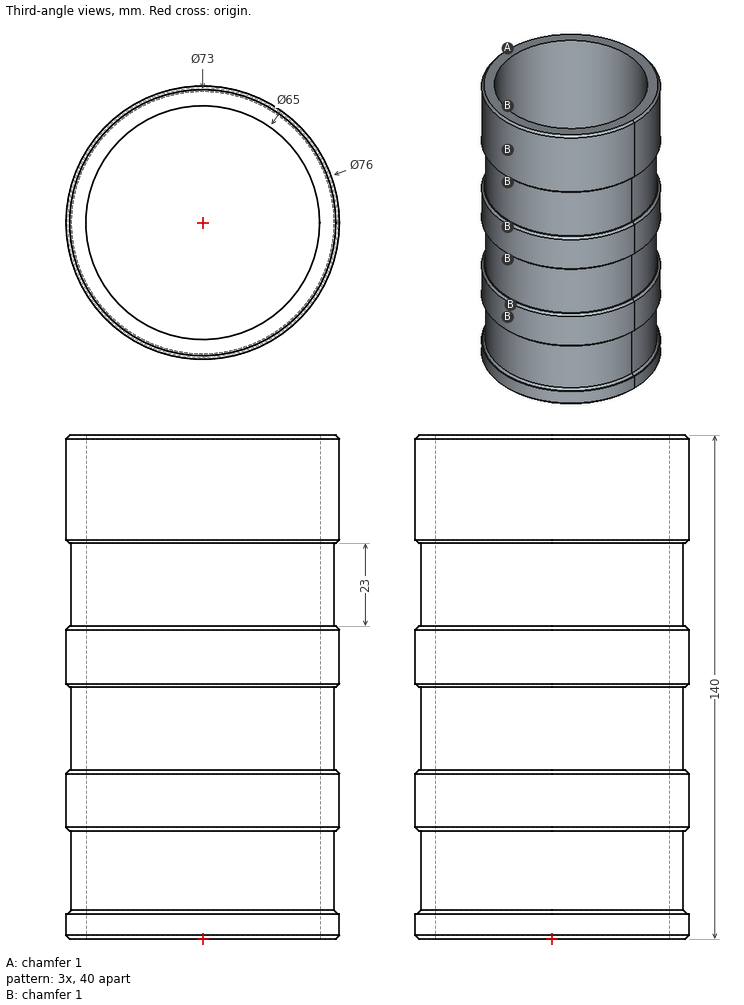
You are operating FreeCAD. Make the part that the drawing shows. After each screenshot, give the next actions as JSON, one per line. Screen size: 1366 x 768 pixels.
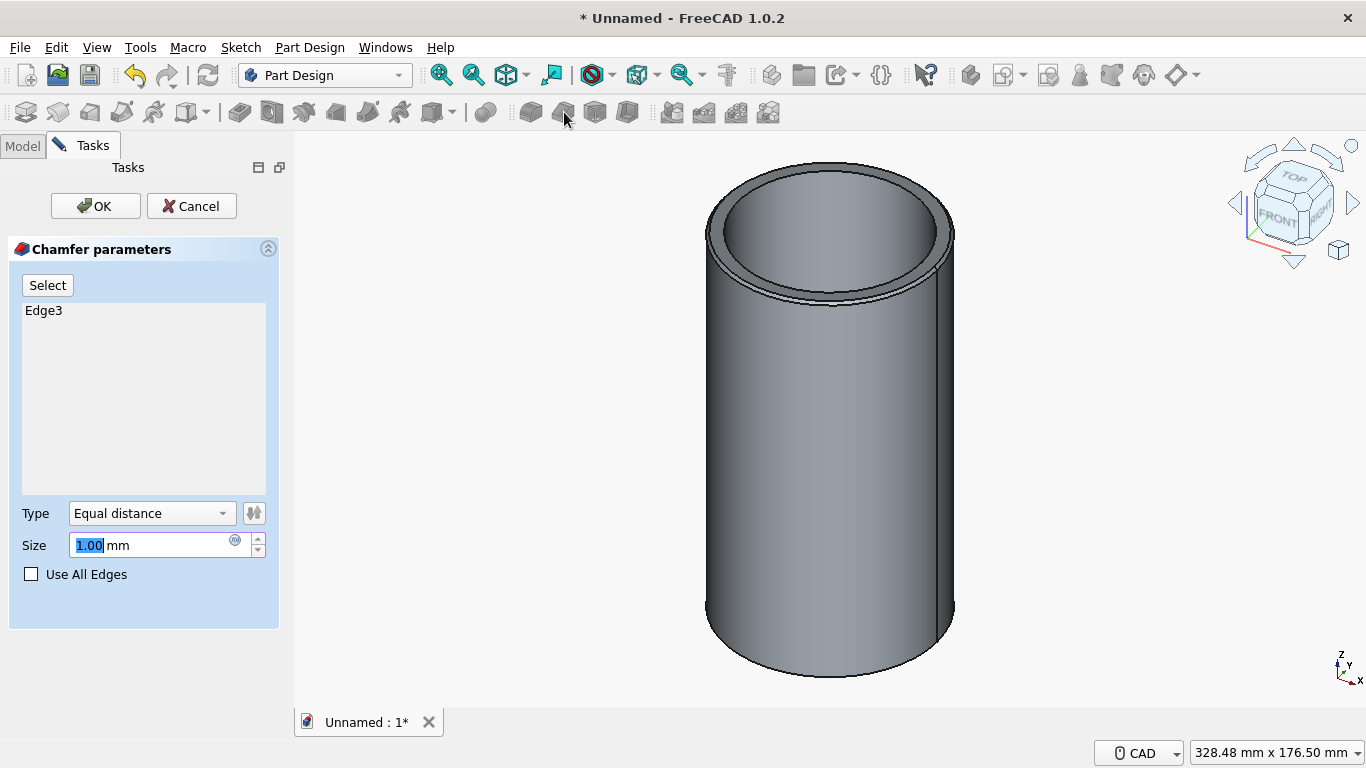
{"action": "type", "text": "1"}
{"action": "key", "text": "Tab"}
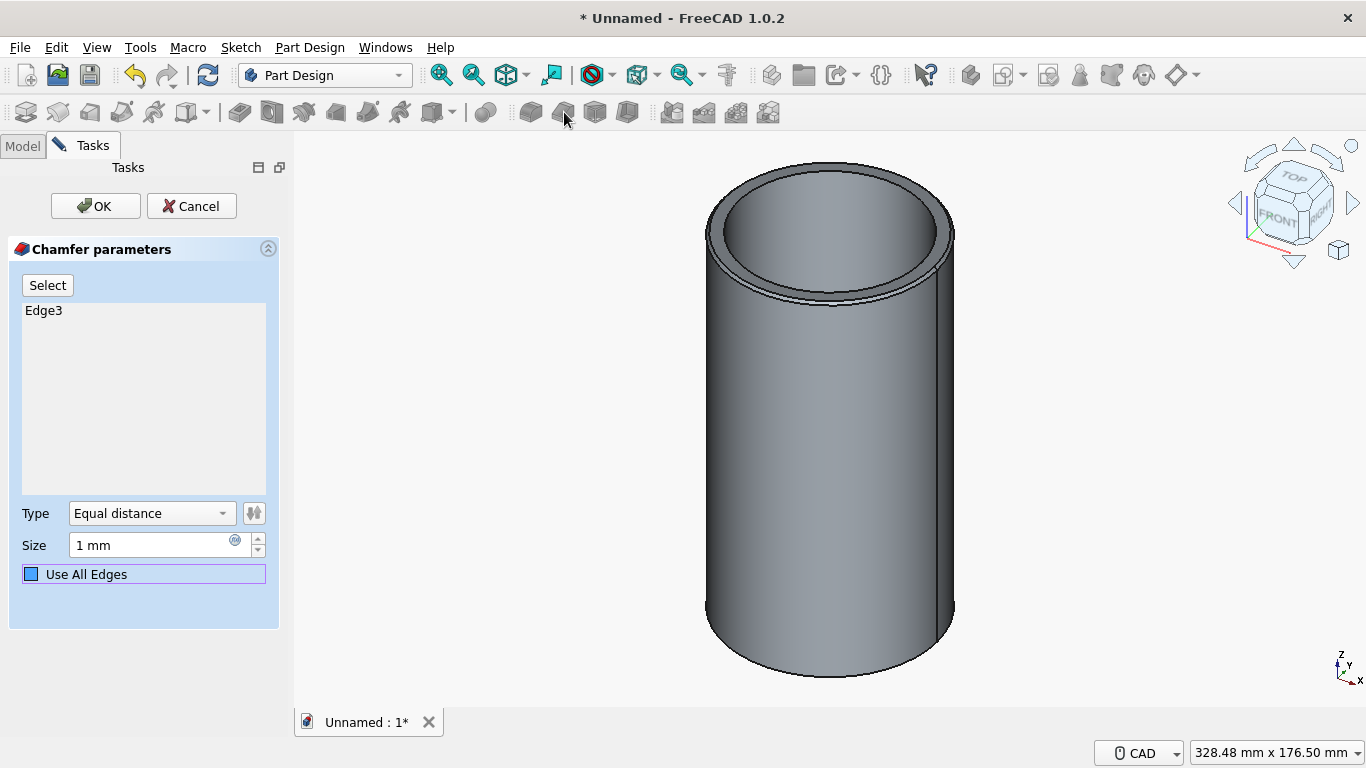
{"action": "left_click", "coordinate": [96, 206]}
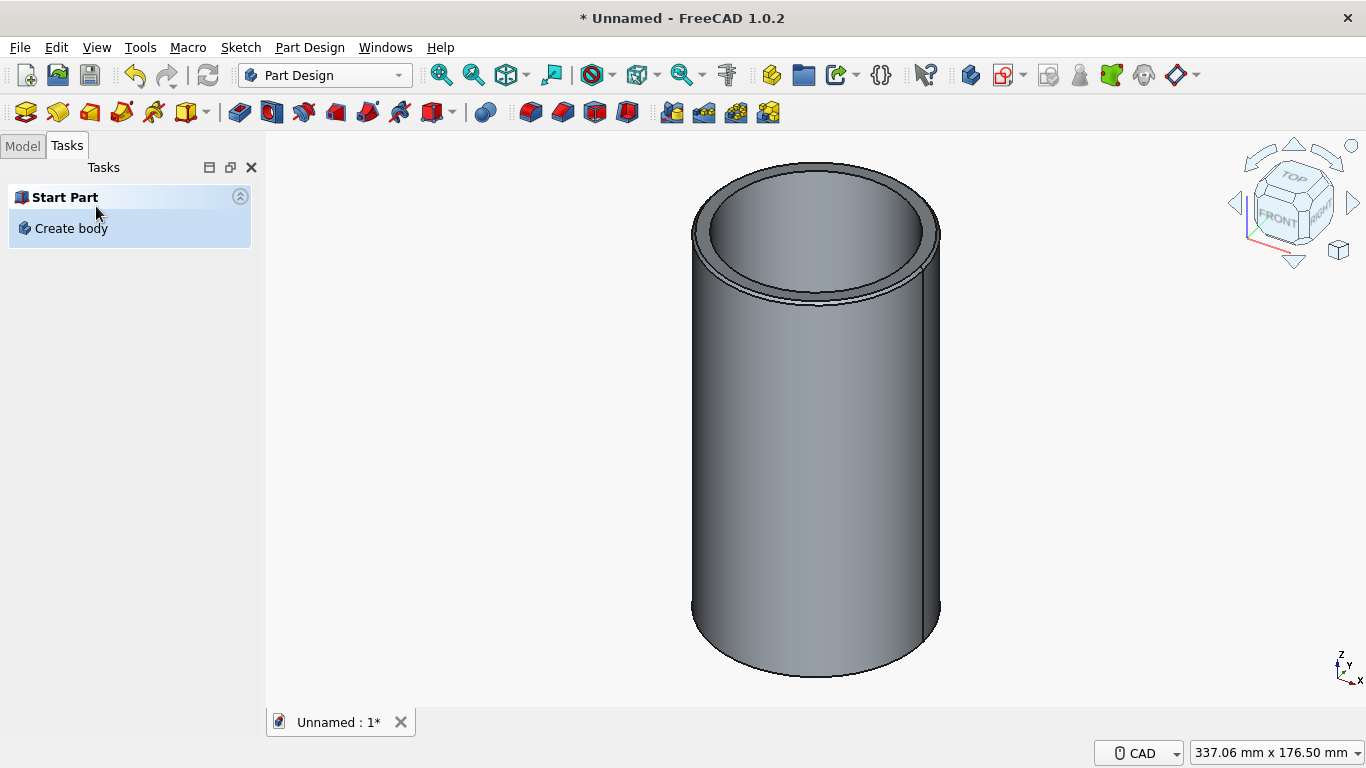
{"action": "left_click", "coordinate": [23, 145]}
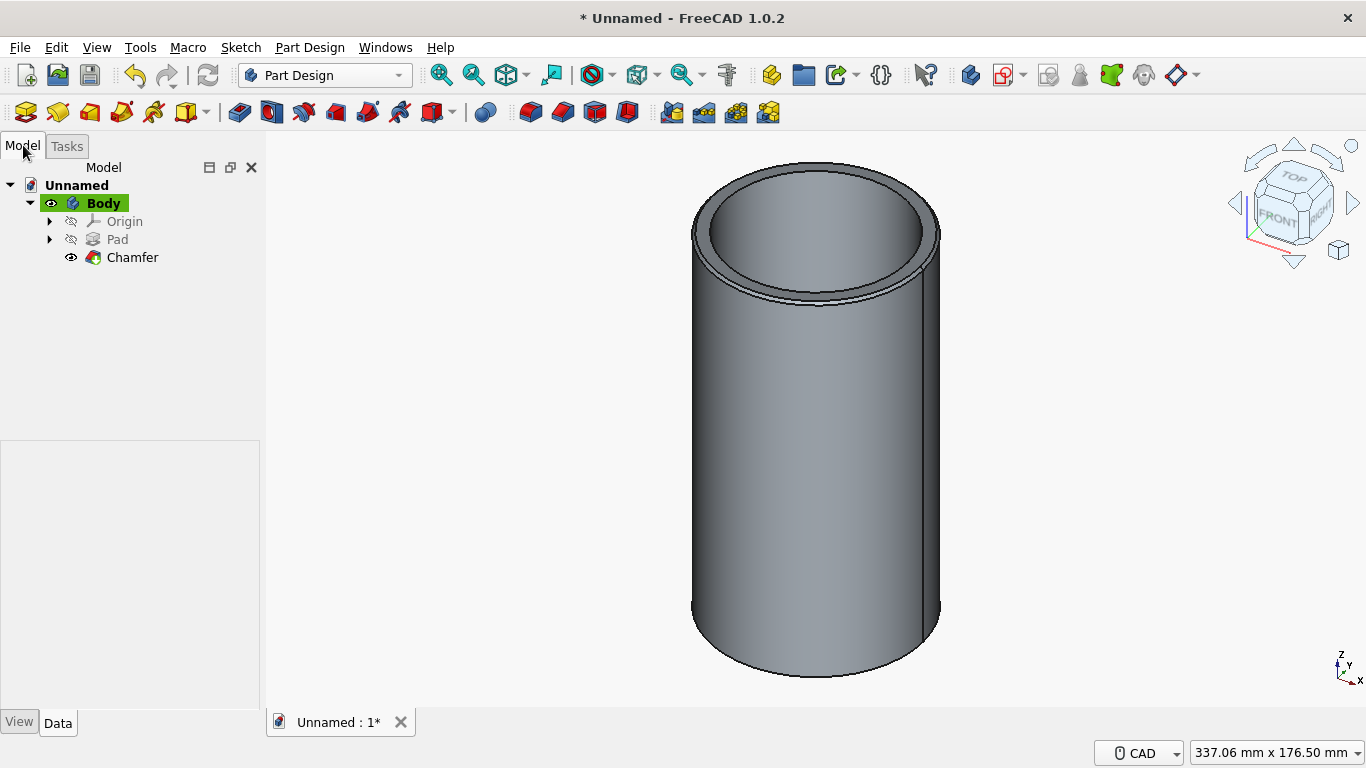
{"action": "left_click", "coordinate": [50, 221]}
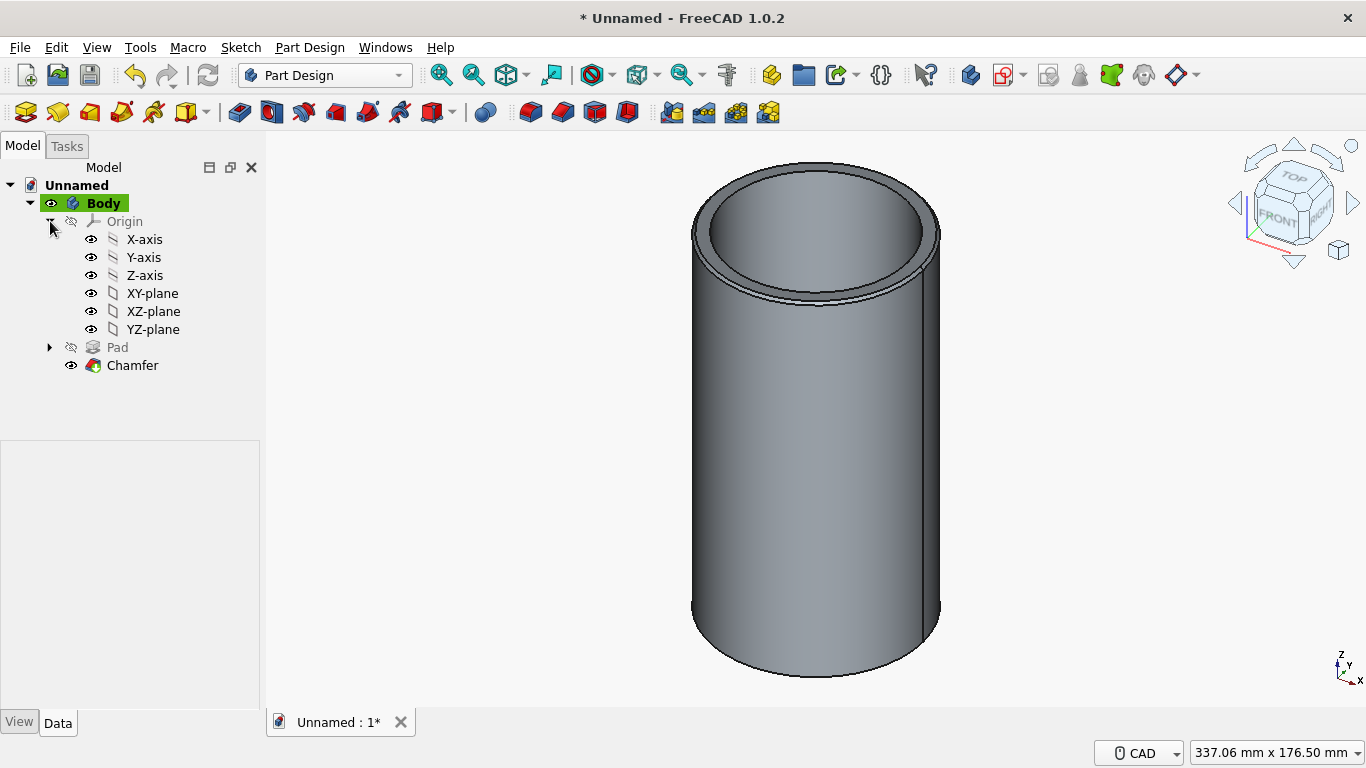
{"action": "left_click", "coordinate": [136, 293]}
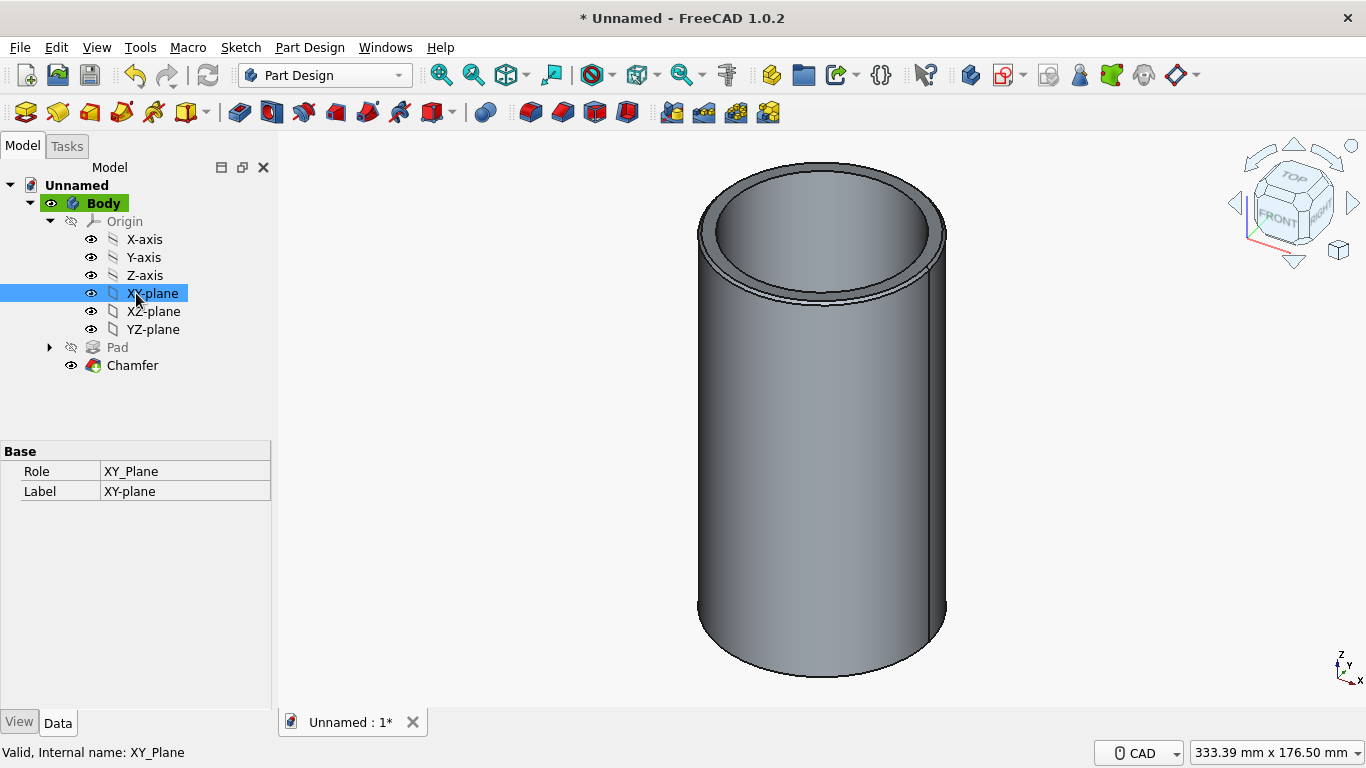
{"action": "left_click", "coordinate": [1176, 76]}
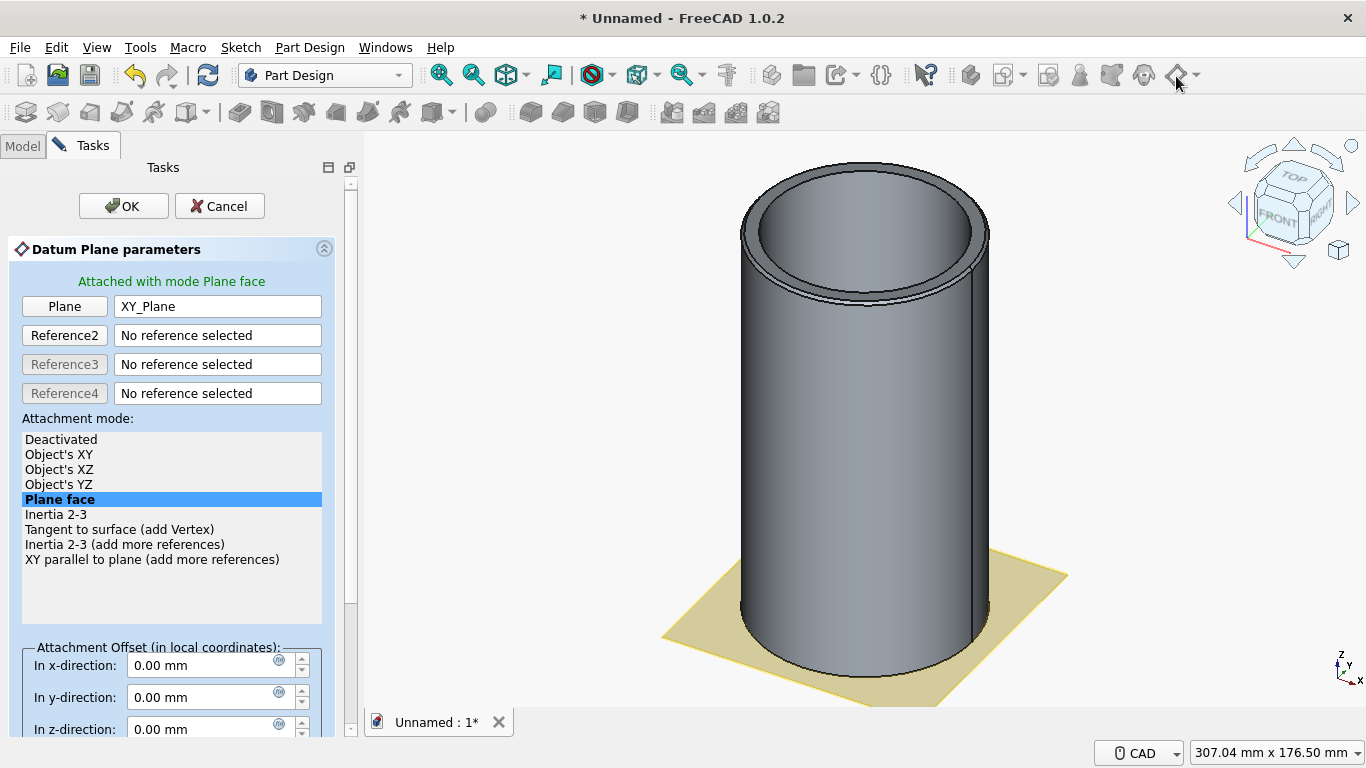
{"action": "scroll", "coordinate": [351, 456], "scroll_direction": "down", "scroll_amount": 2}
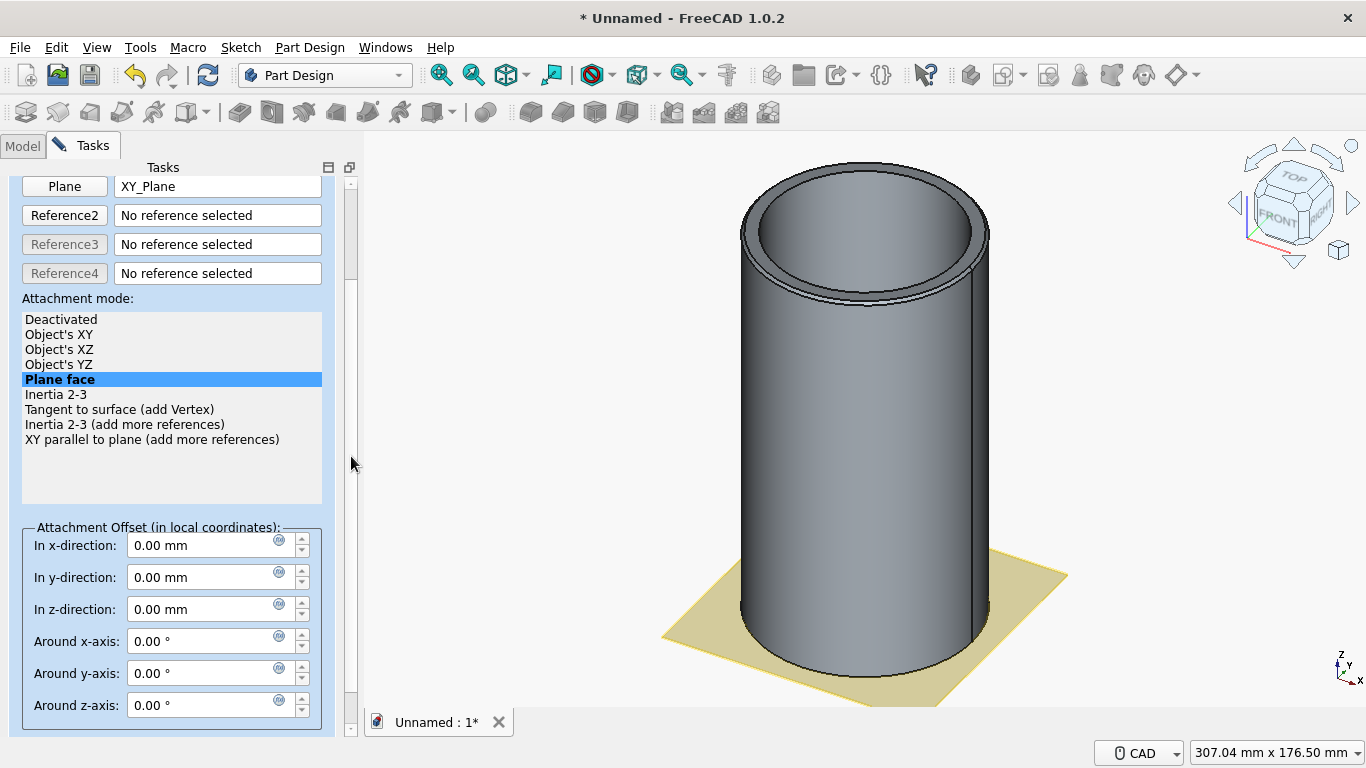
{"action": "triple_click", "coordinate": [210, 609]}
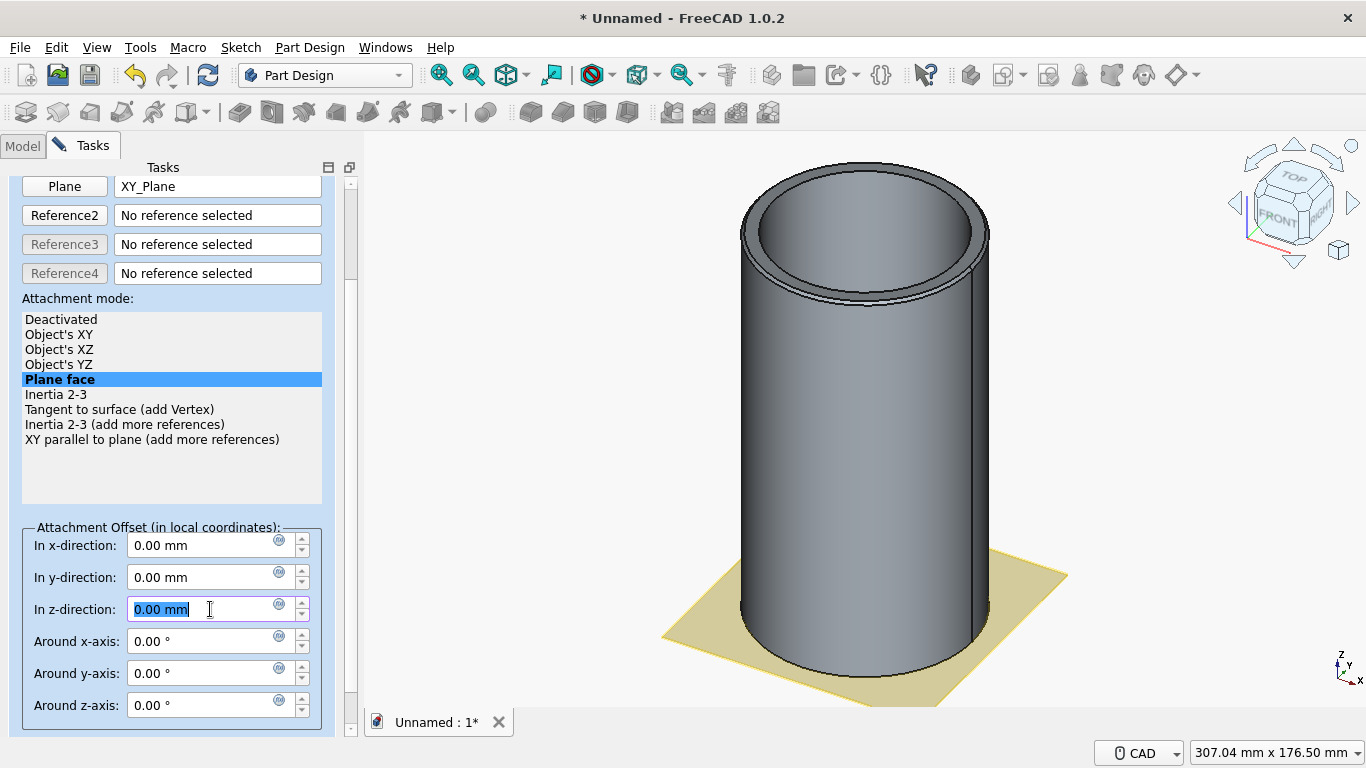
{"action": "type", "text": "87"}
{"action": "key", "text": "Tab"}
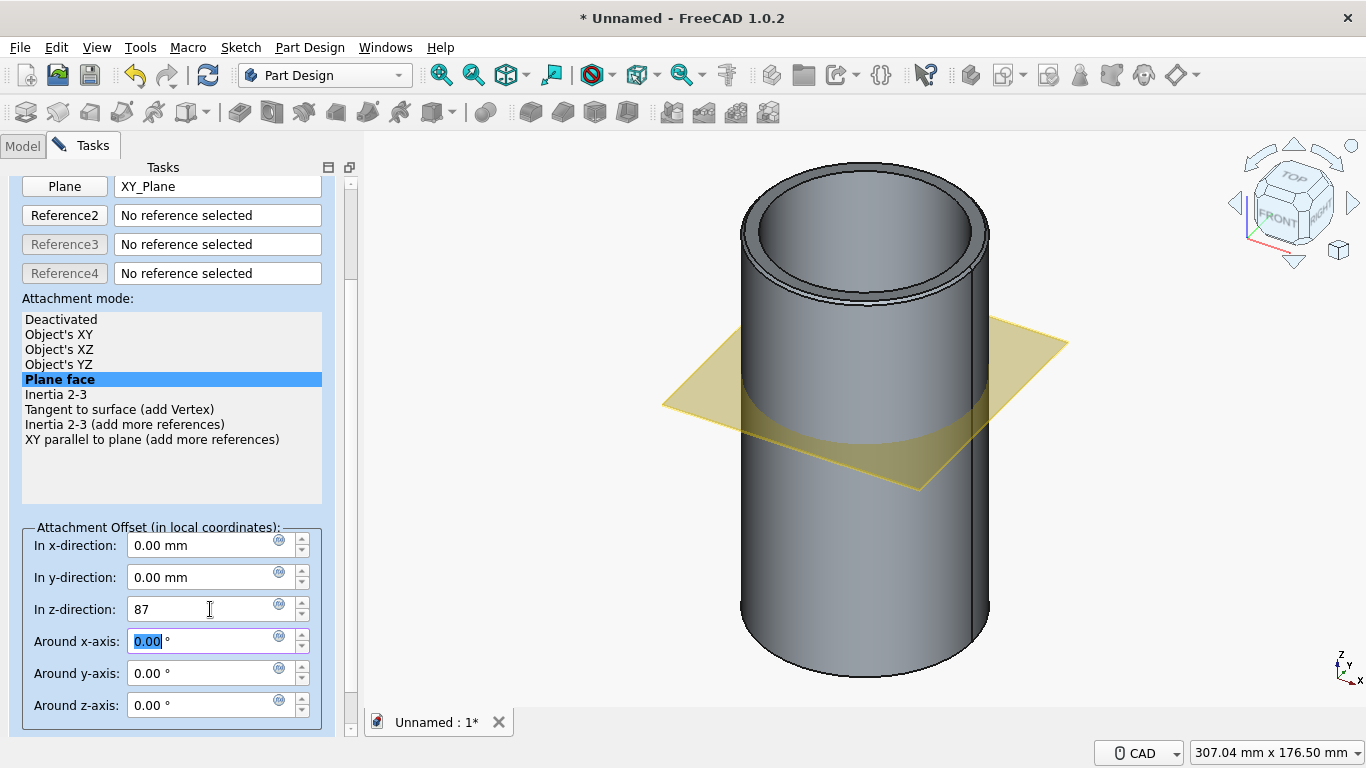
{"action": "scroll", "coordinate": [351, 456], "scroll_direction": "up", "scroll_amount": 3}